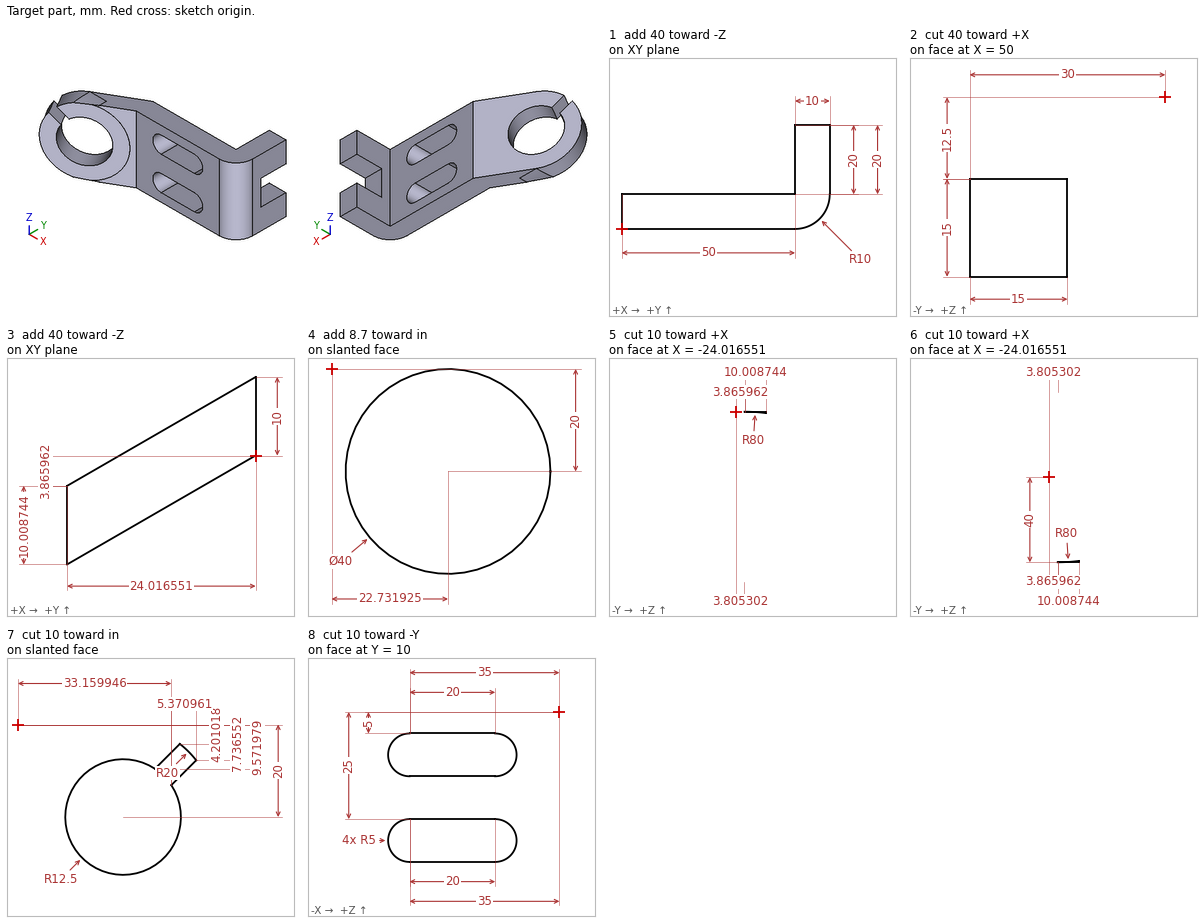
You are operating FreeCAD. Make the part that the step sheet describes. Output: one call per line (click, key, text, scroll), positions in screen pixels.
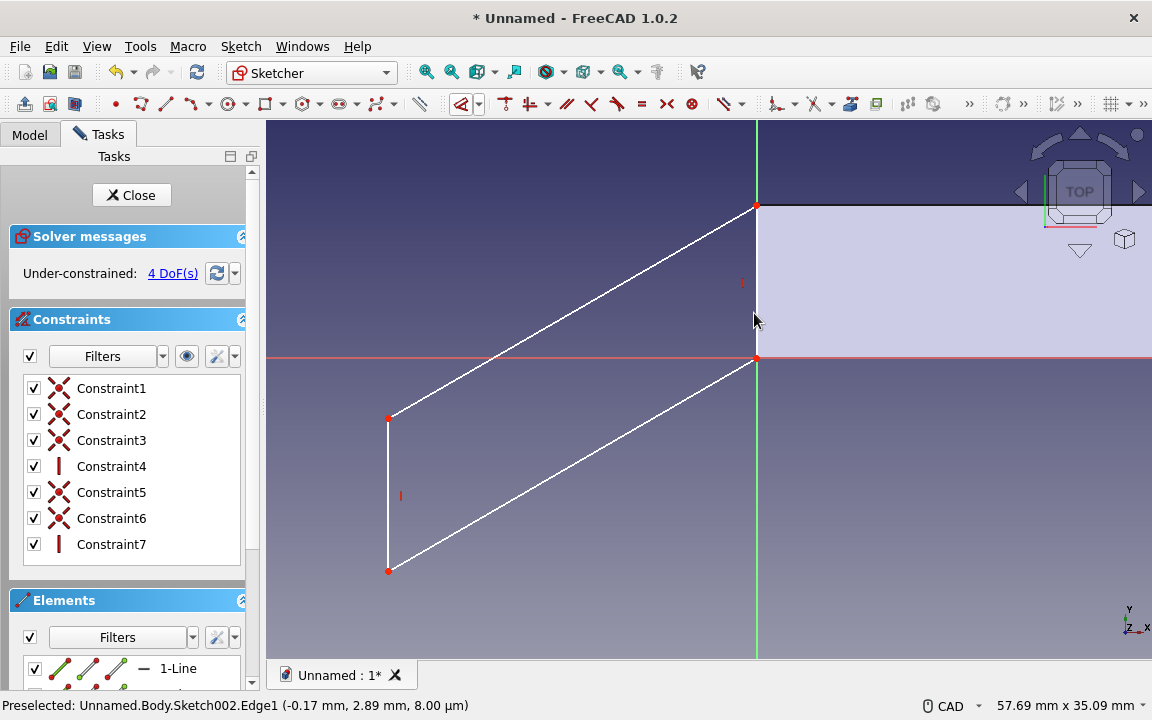
click(757, 313)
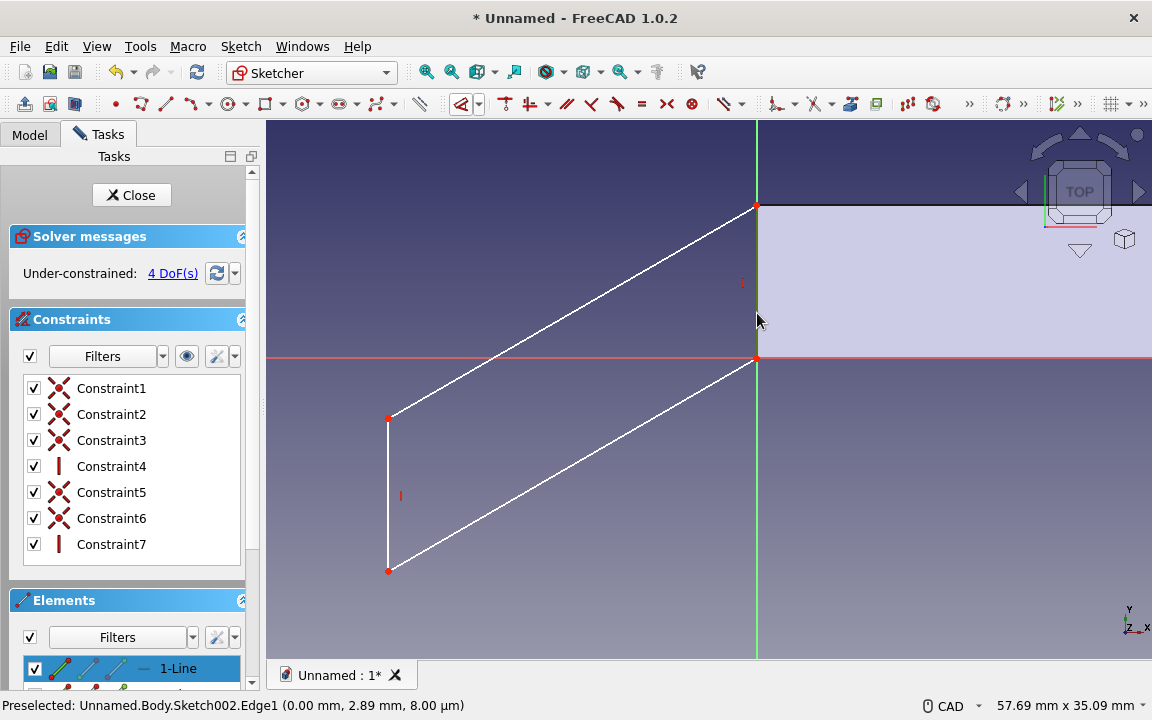
click(478, 104)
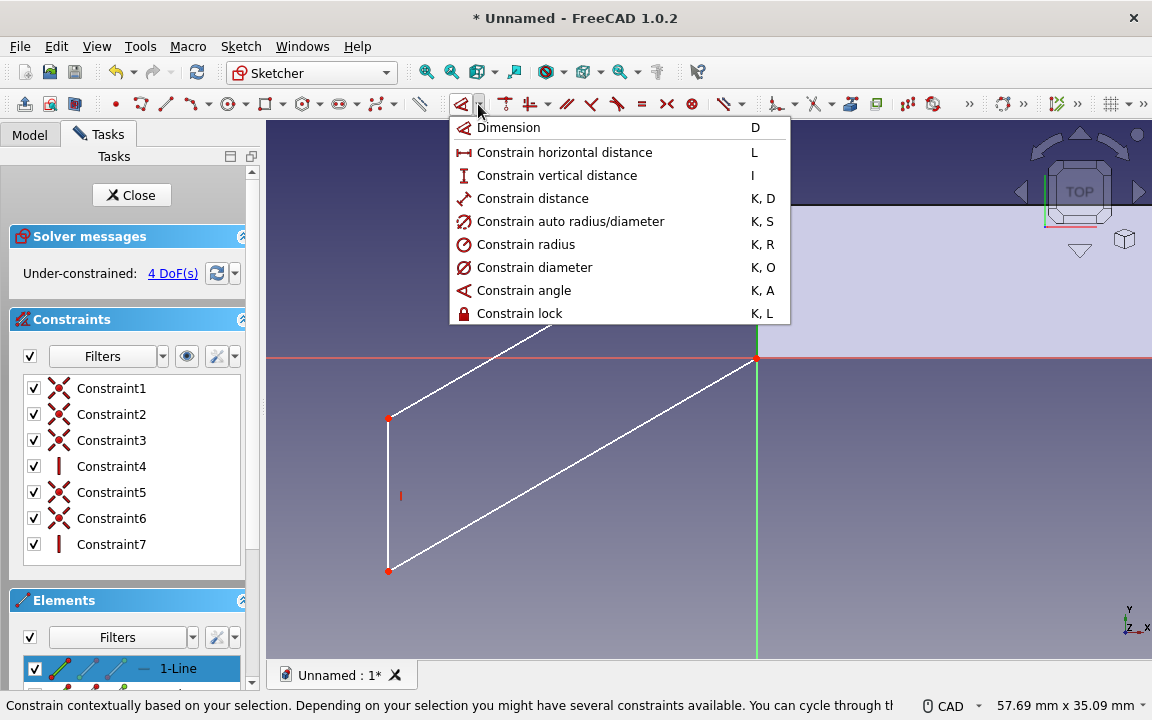
click(620, 176)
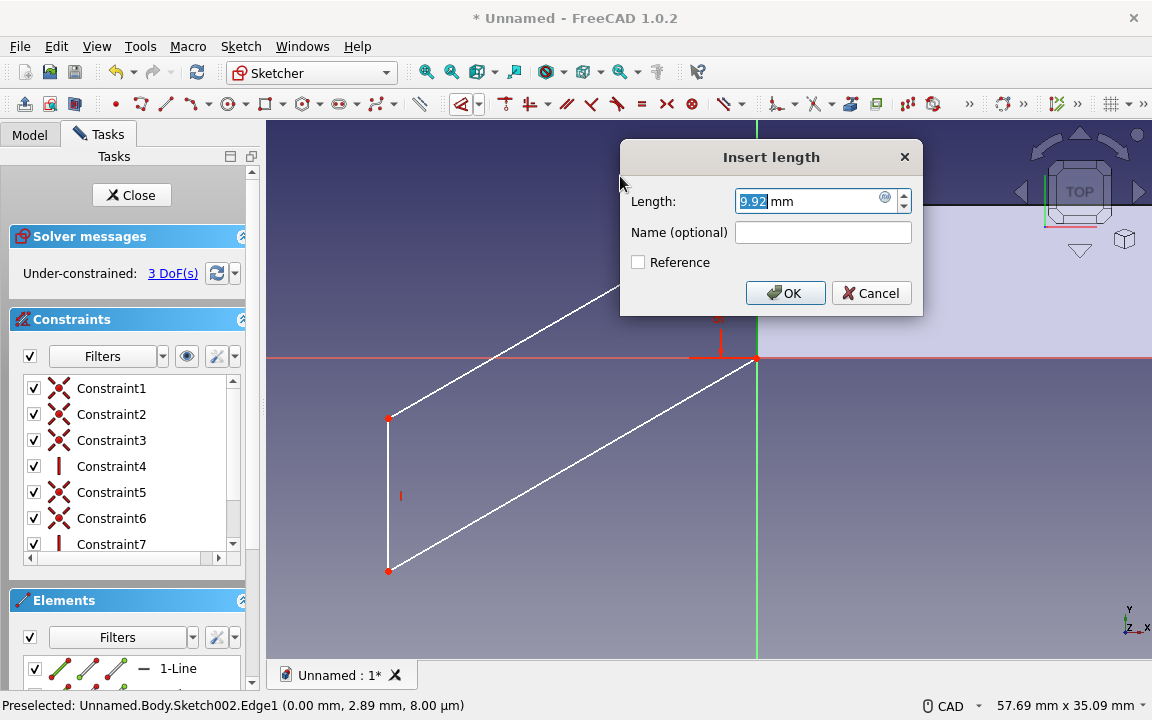
text(10)
key(Return)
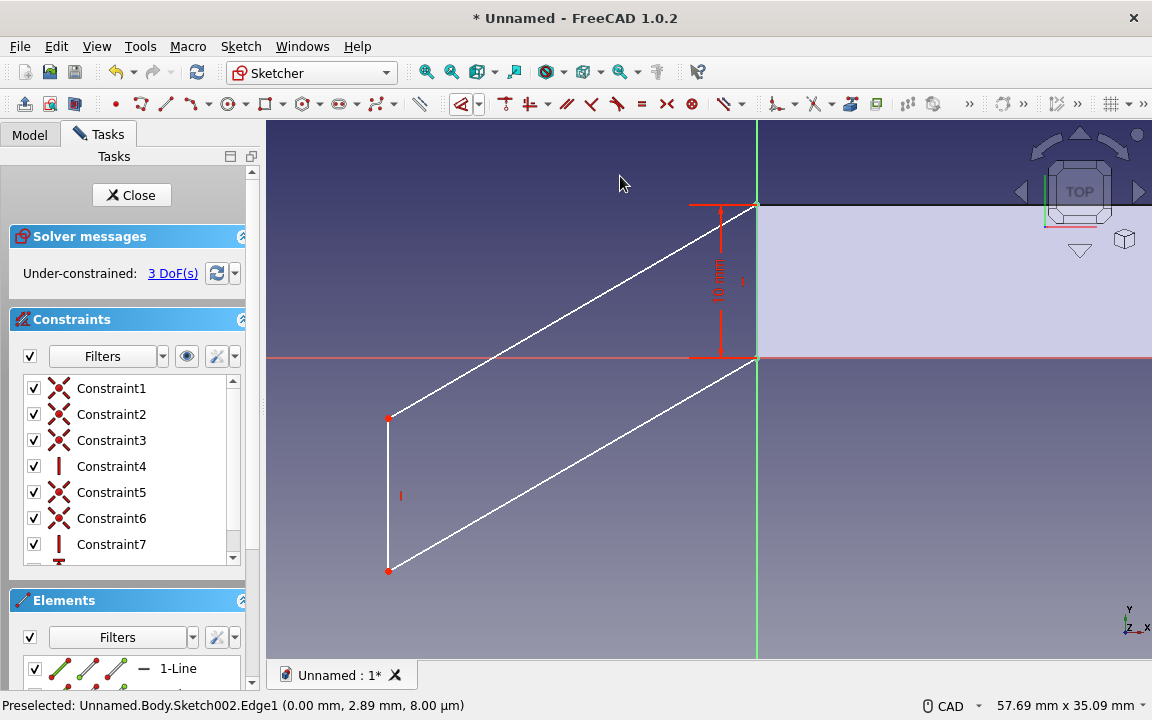
click(388, 465)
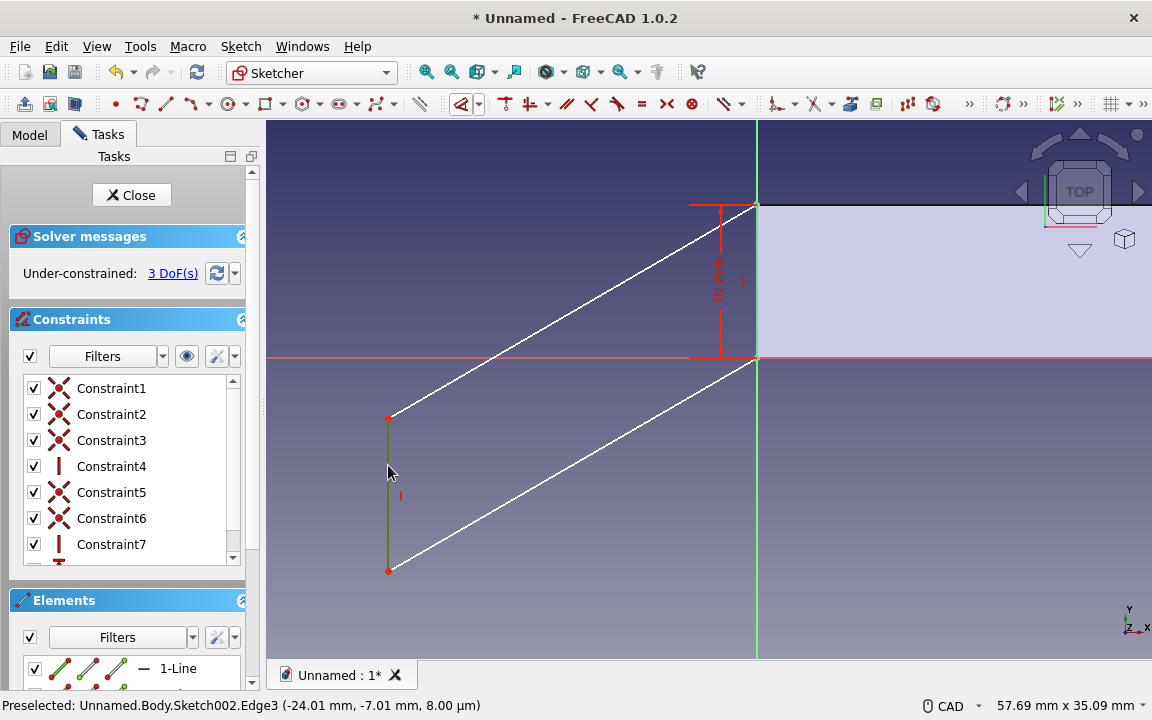
key(i)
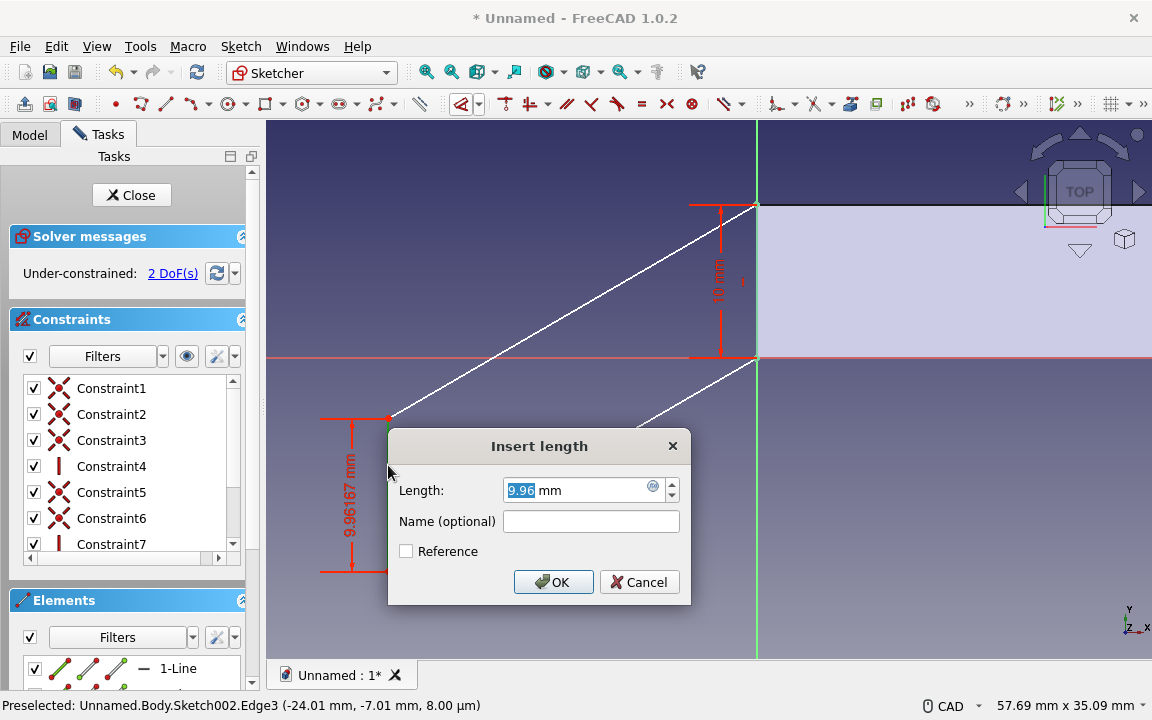
text(10.008744)
key(Return)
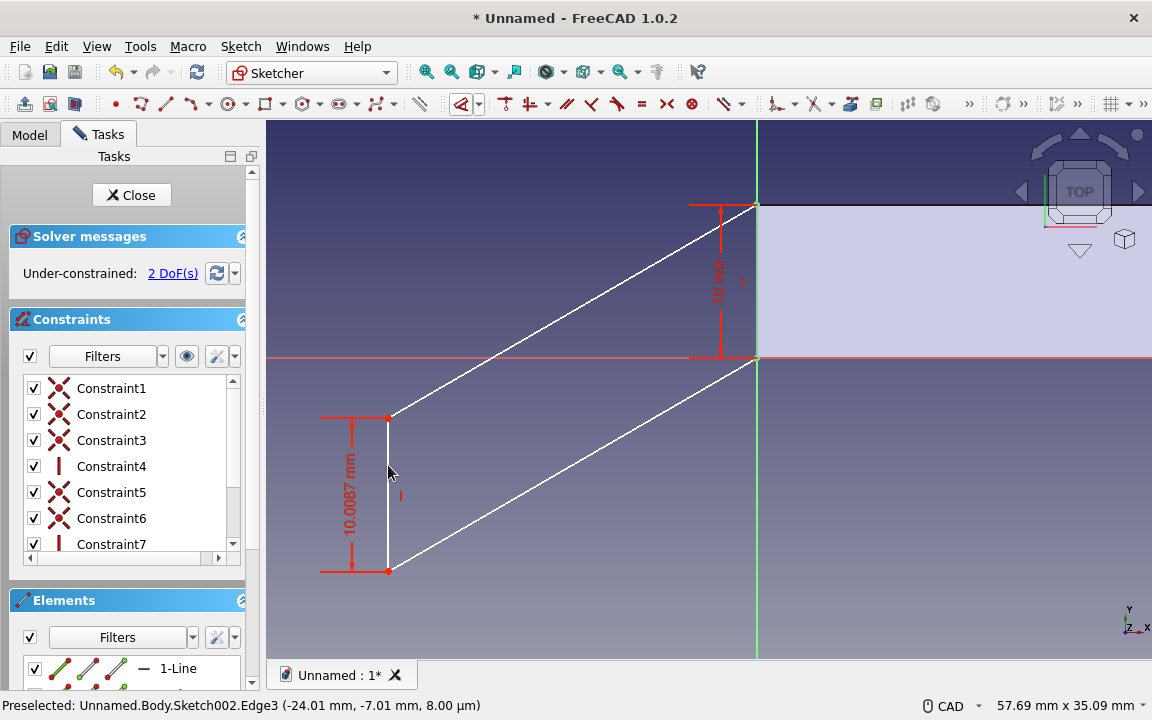
click(388, 418)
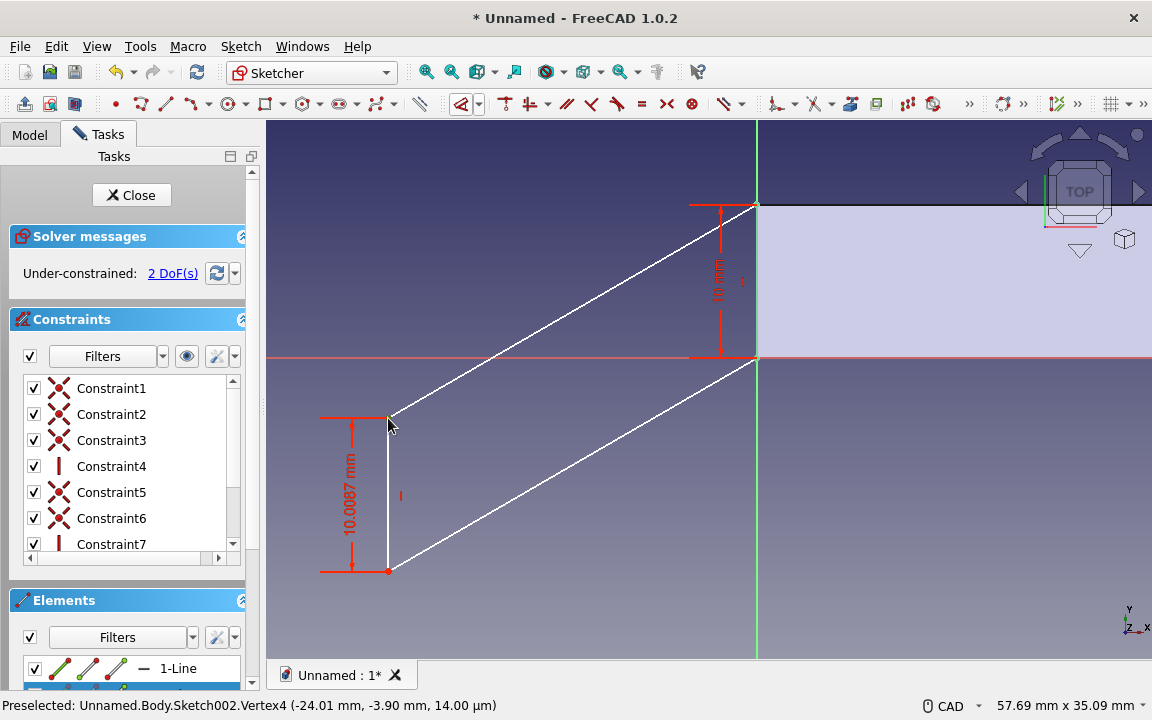
click(478, 104)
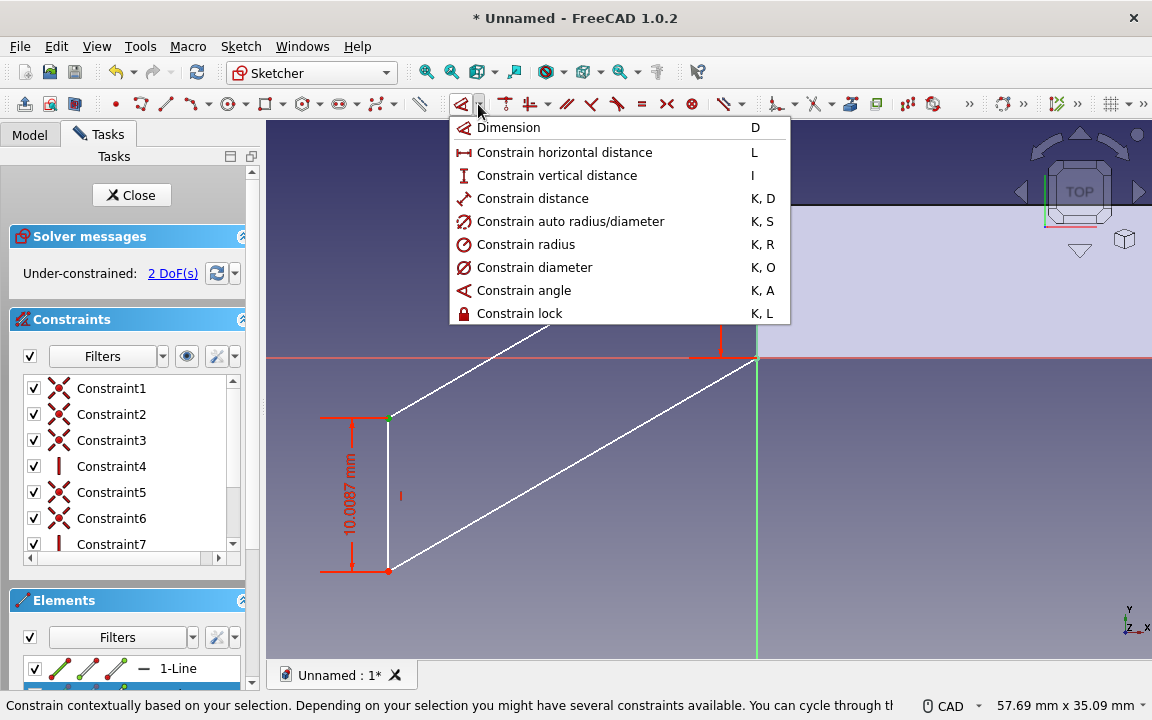
click(620, 176)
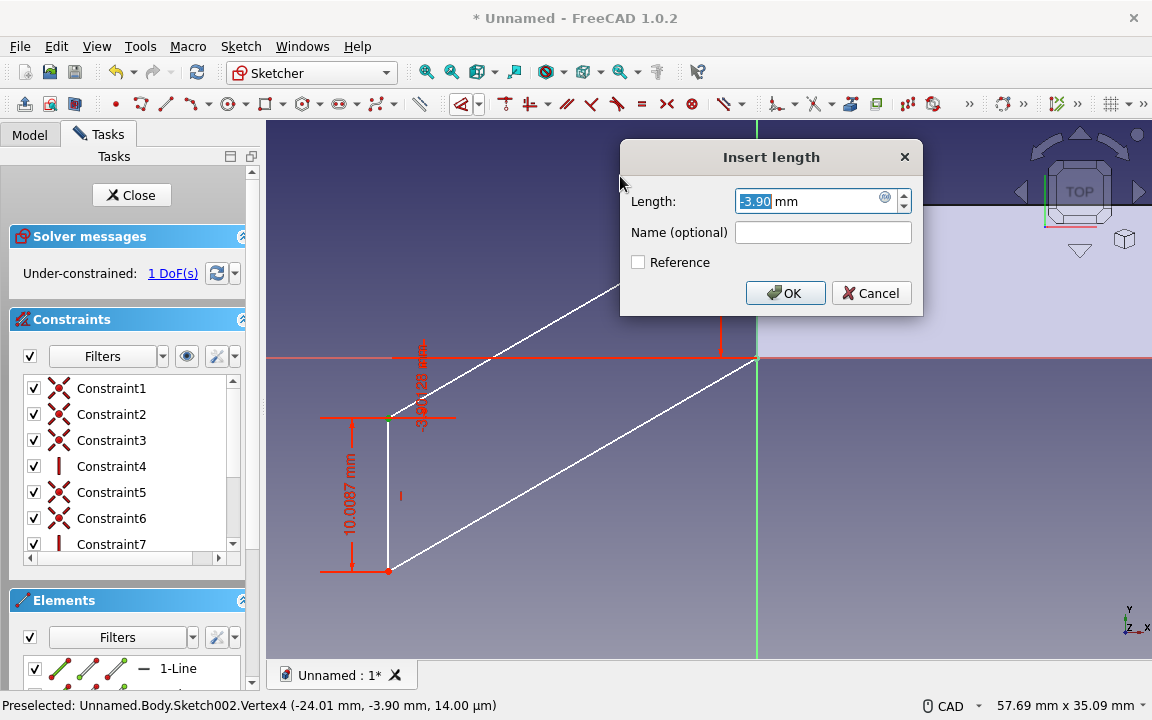
text(-3.865962)
key(Return)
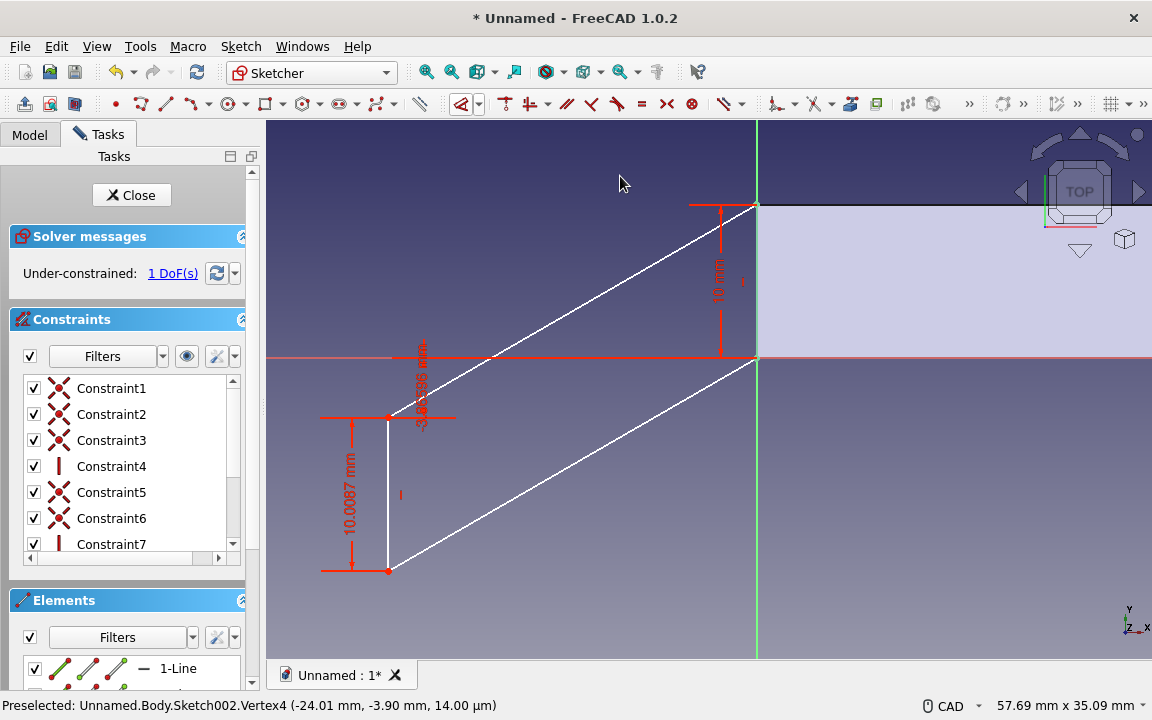
click(388, 418)